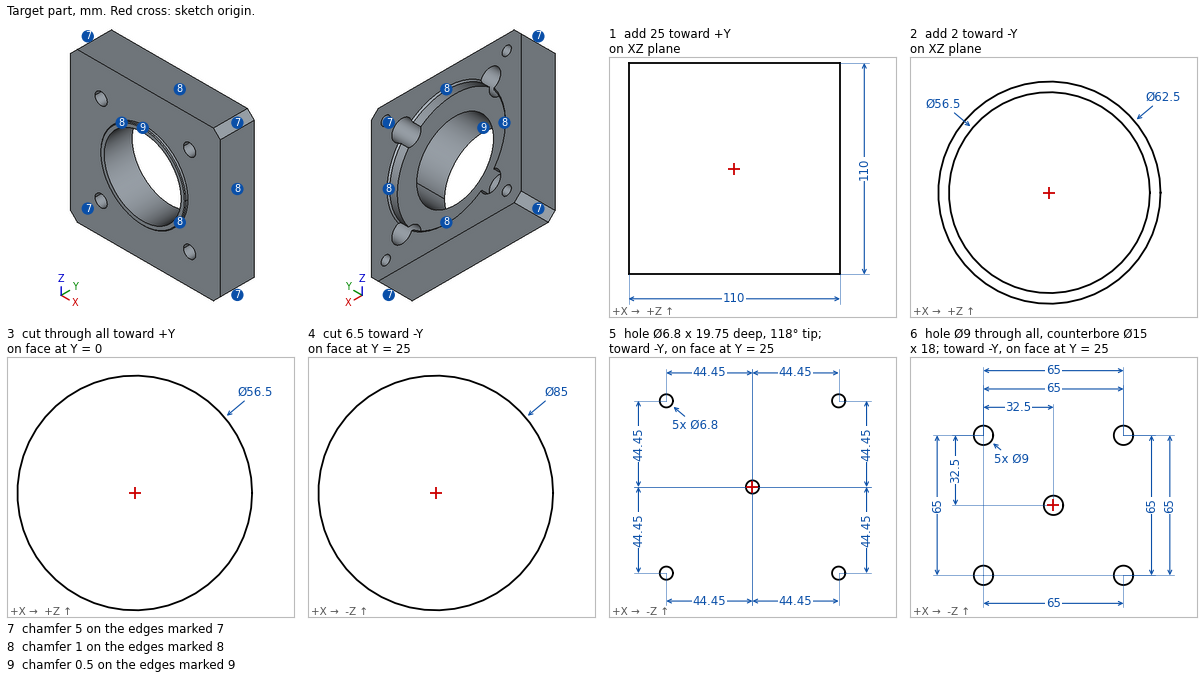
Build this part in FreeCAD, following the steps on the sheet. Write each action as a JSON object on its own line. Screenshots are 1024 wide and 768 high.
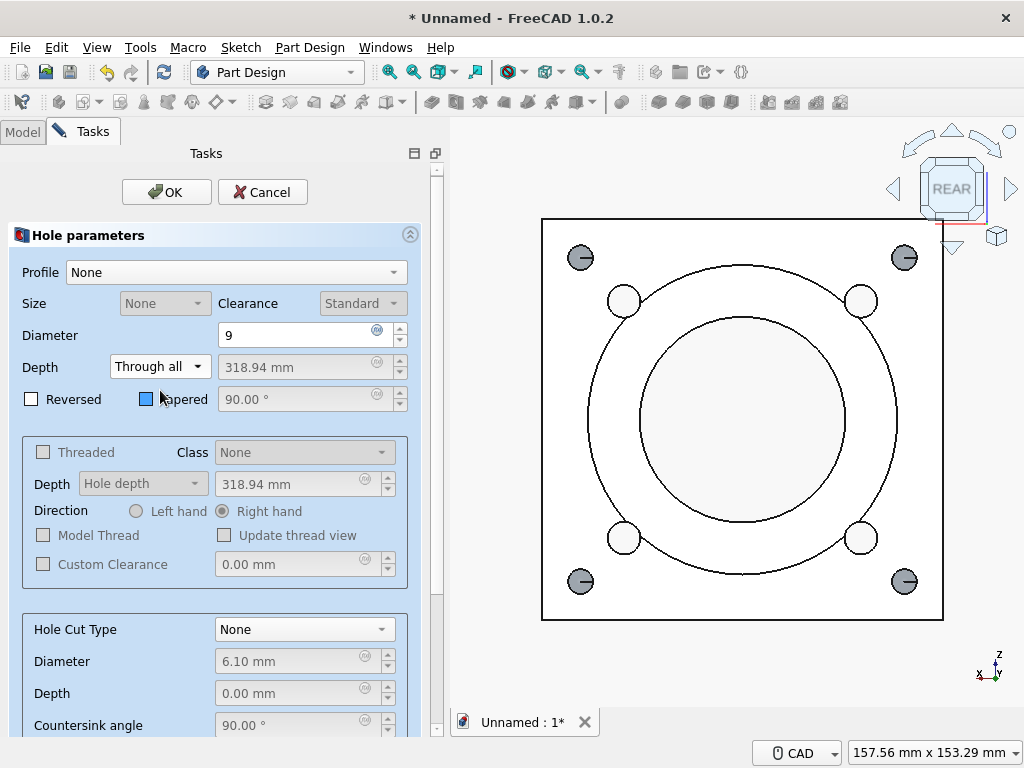
{"action": "left_click", "coordinate": [306, 630]}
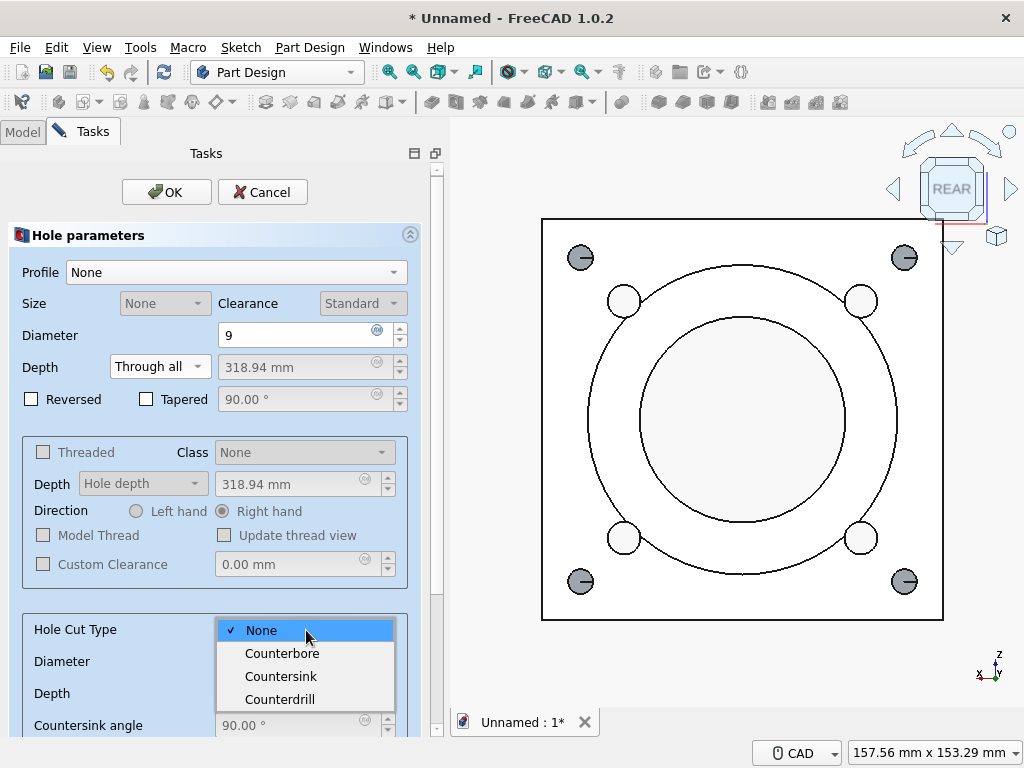
{"action": "left_click", "coordinate": [304, 654]}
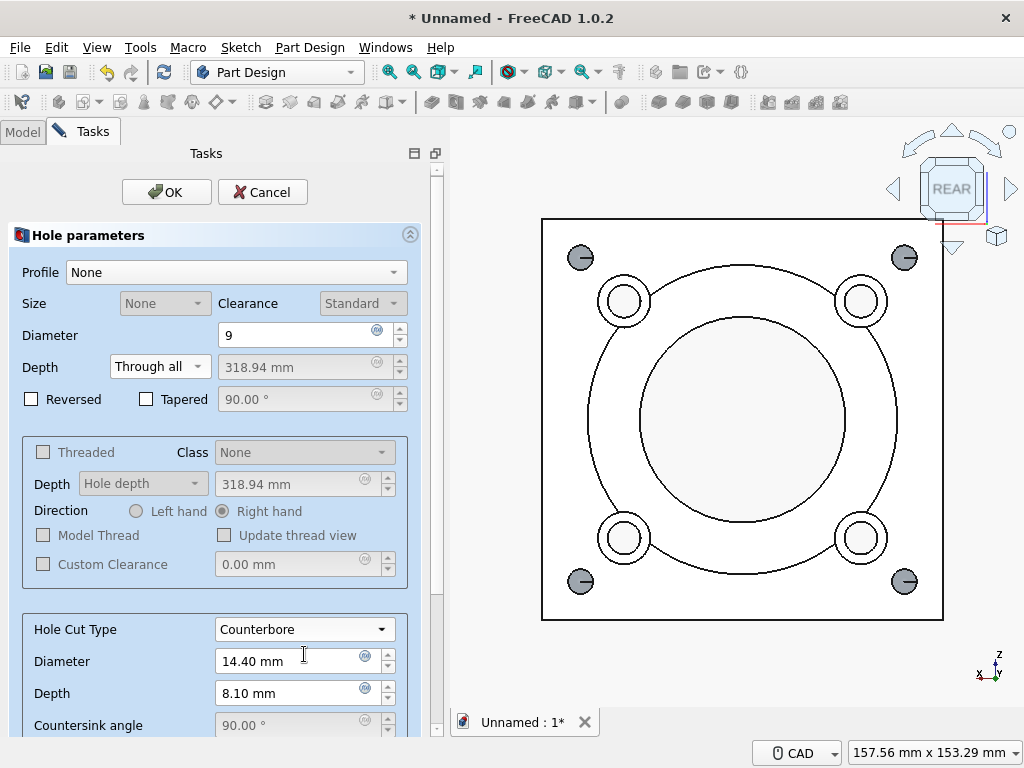
{"action": "triple_click", "coordinate": [298, 661]}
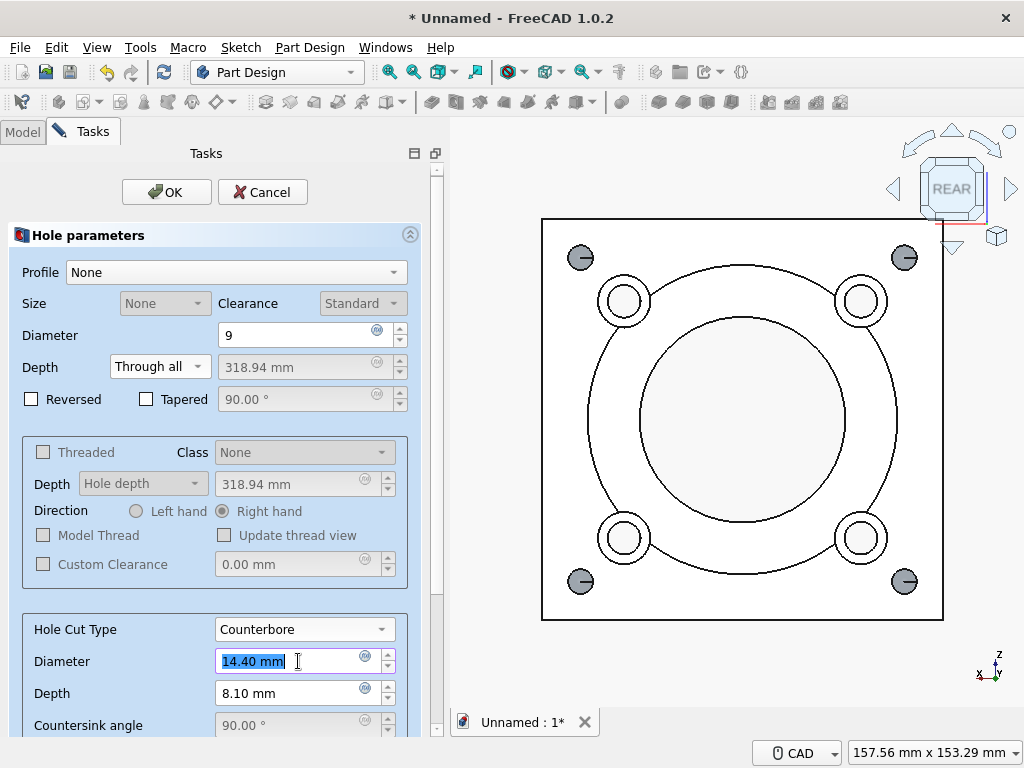
{"action": "type", "text": "15"}
{"action": "key", "text": "Tab"}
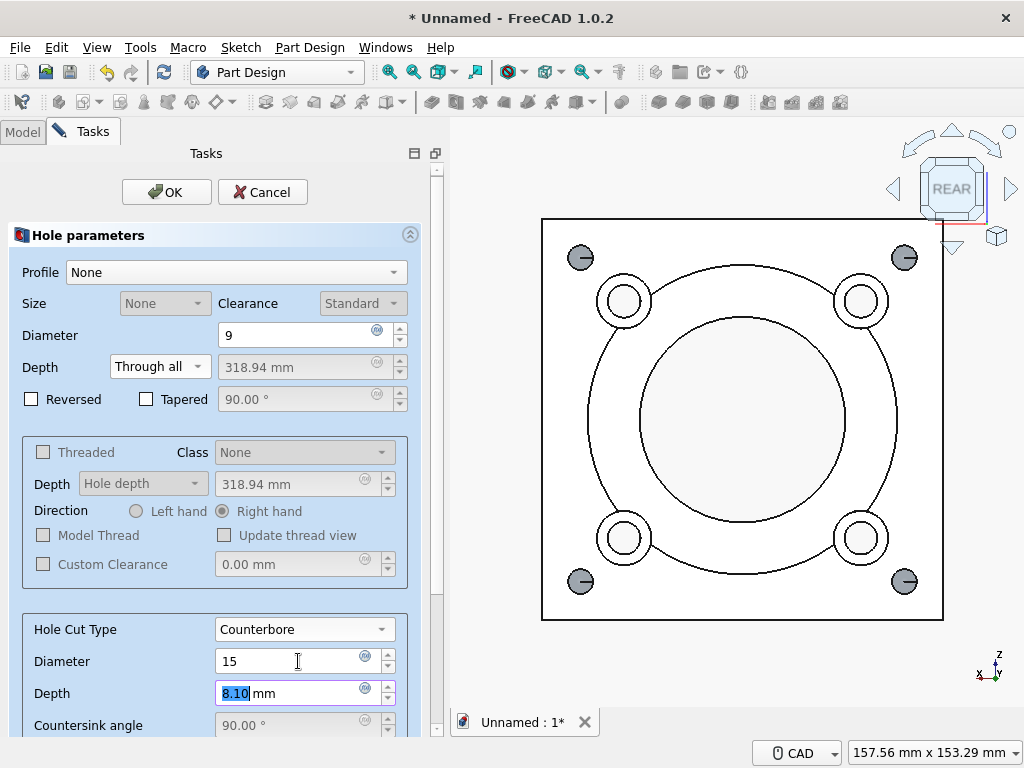
{"action": "type", "text": "18"}
{"action": "key", "text": "Tab"}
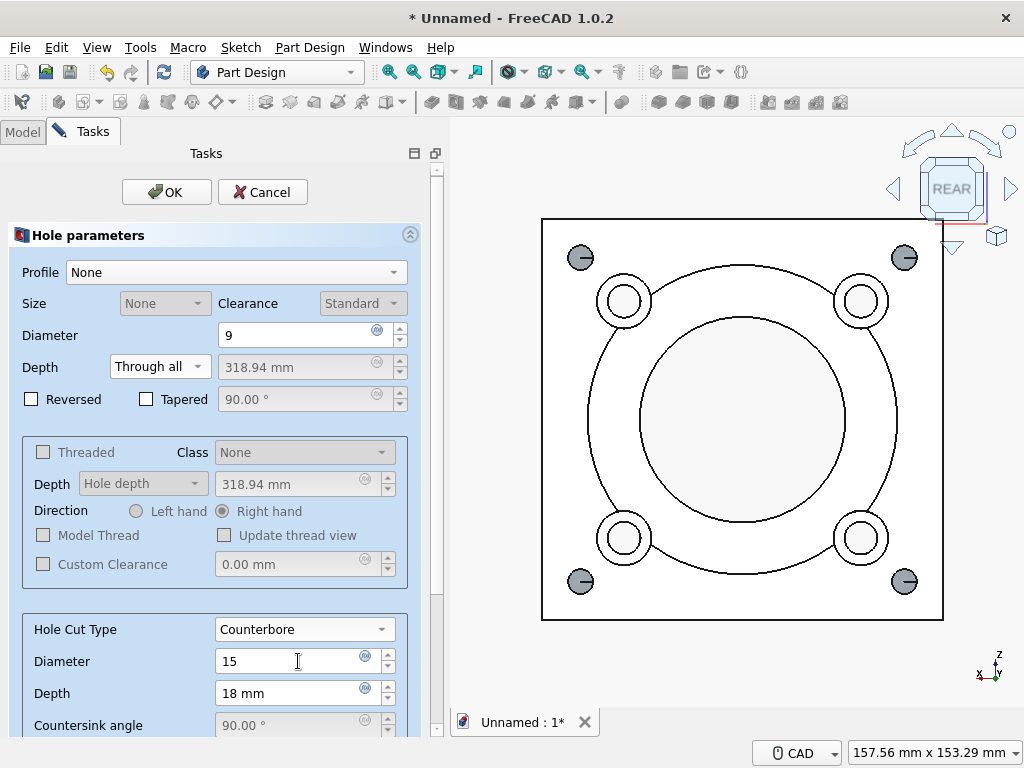
{"action": "left_click", "coordinate": [167, 192]}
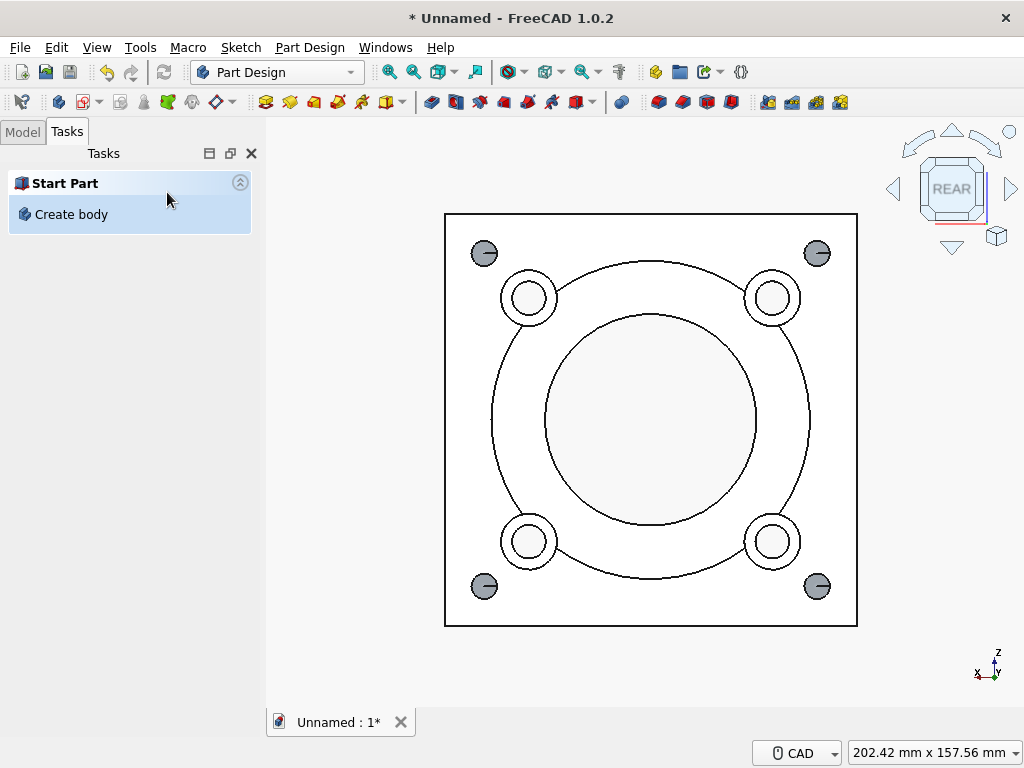
{"action": "key", "text": "0"}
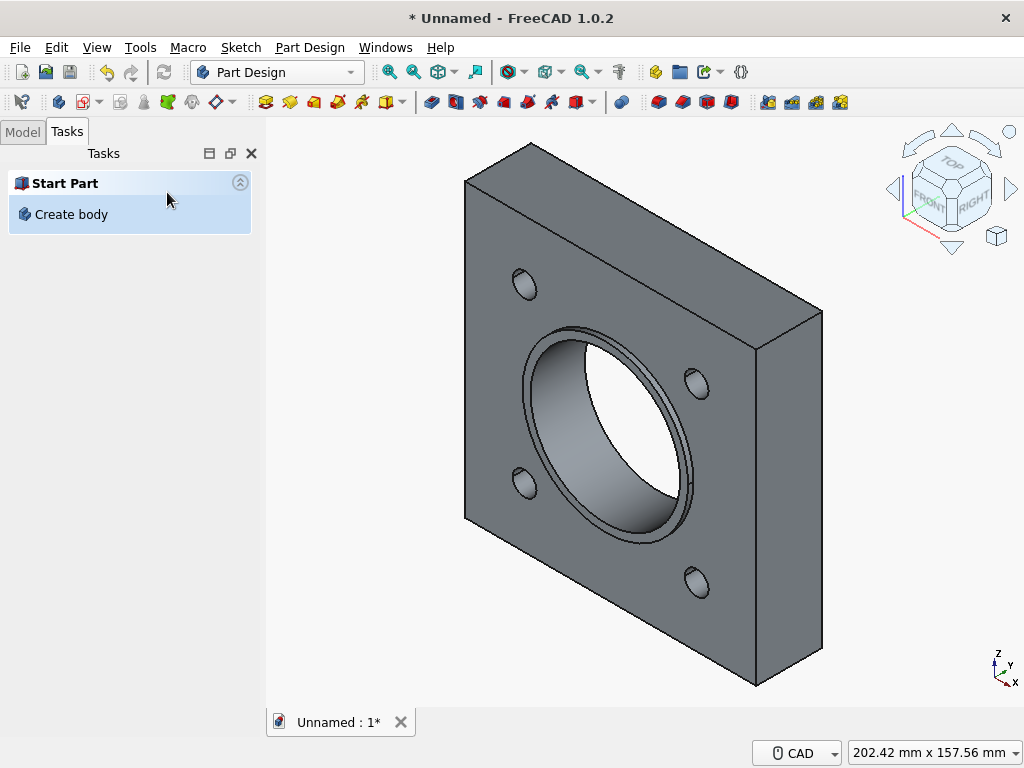
{"action": "left_click", "coordinate": [789, 329]}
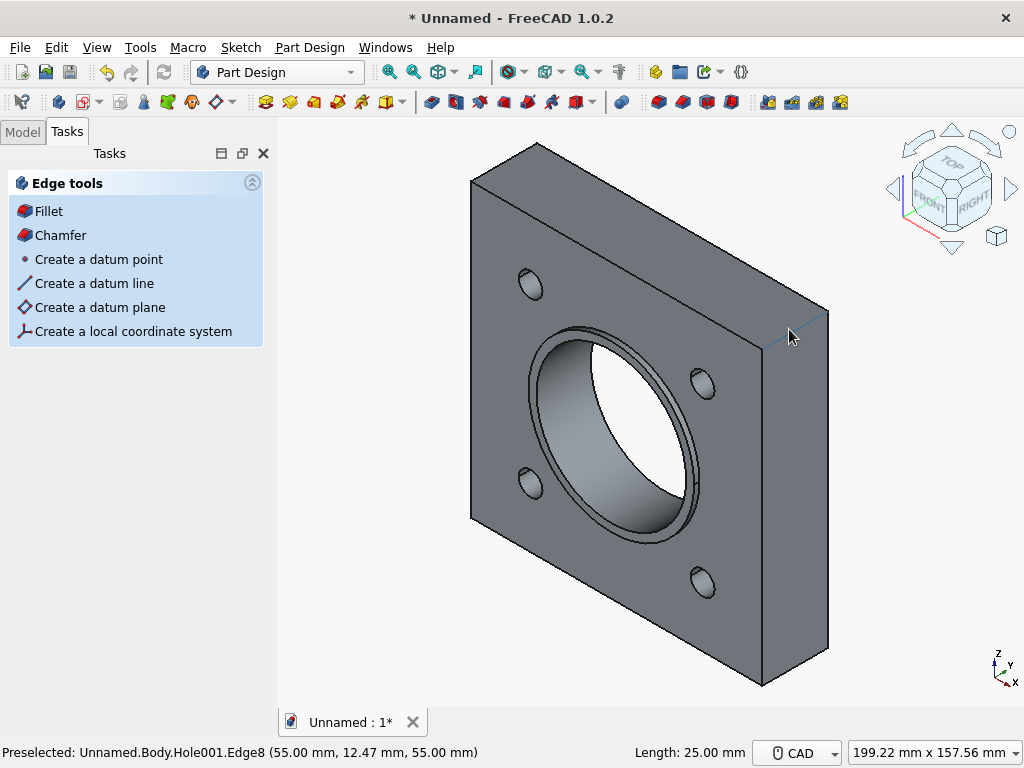
{"action": "key", "text": "2"}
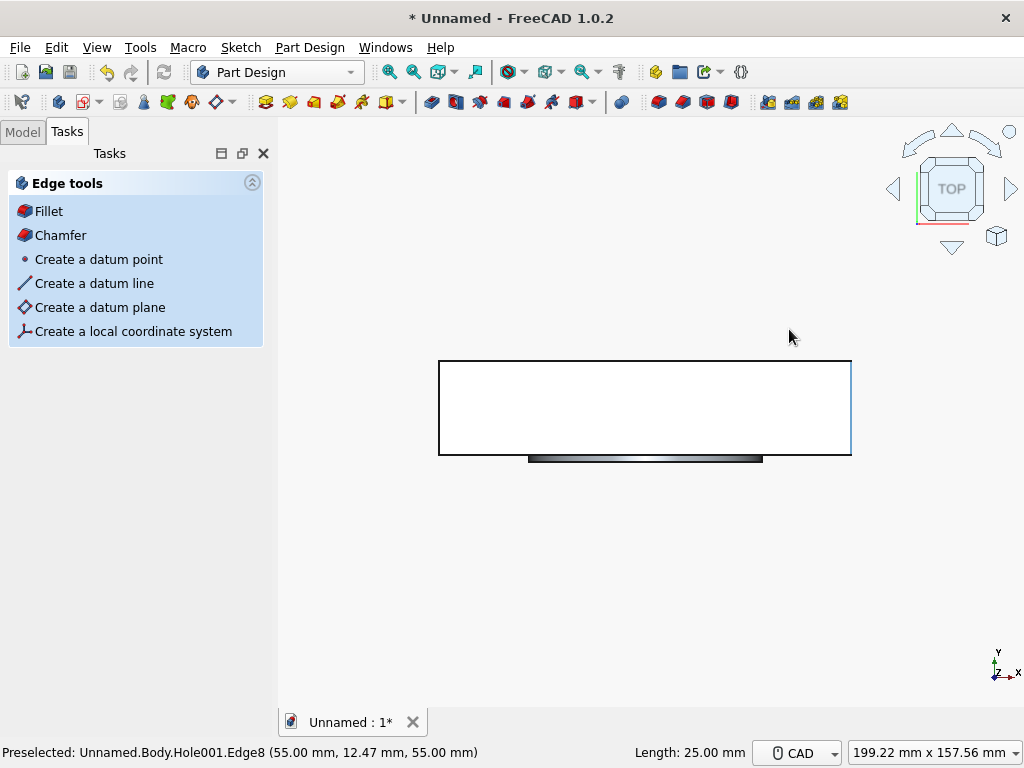
{"action": "left_click", "coordinate": [439, 407], "text": "ctrl"}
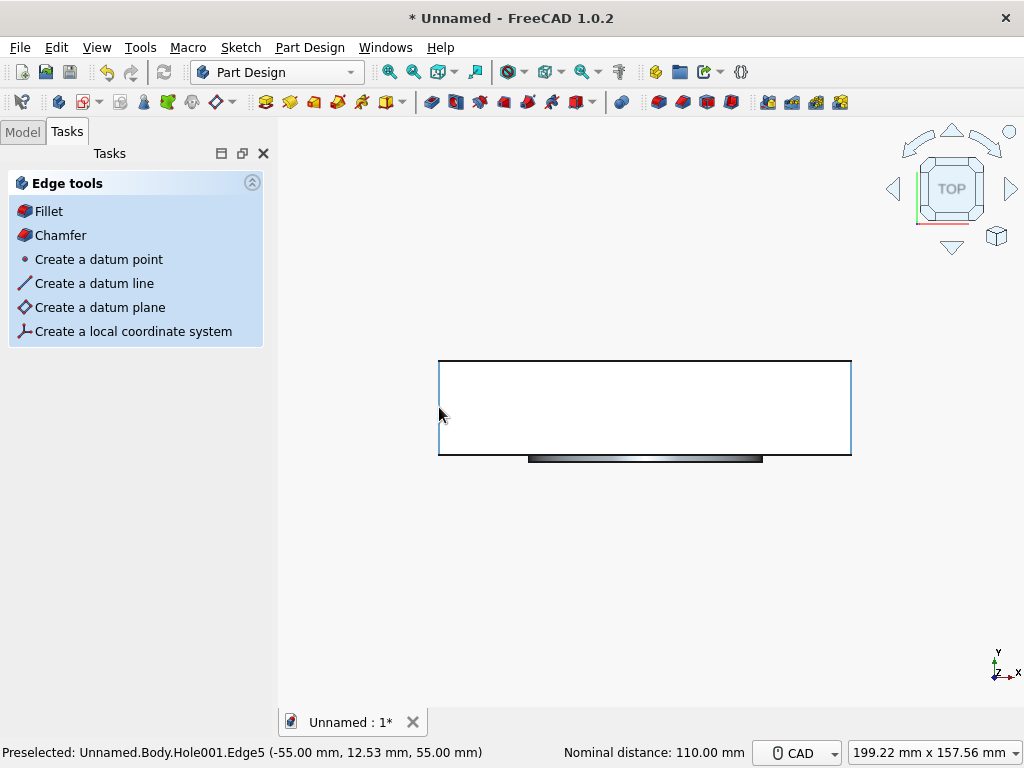
{"action": "key", "text": "1"}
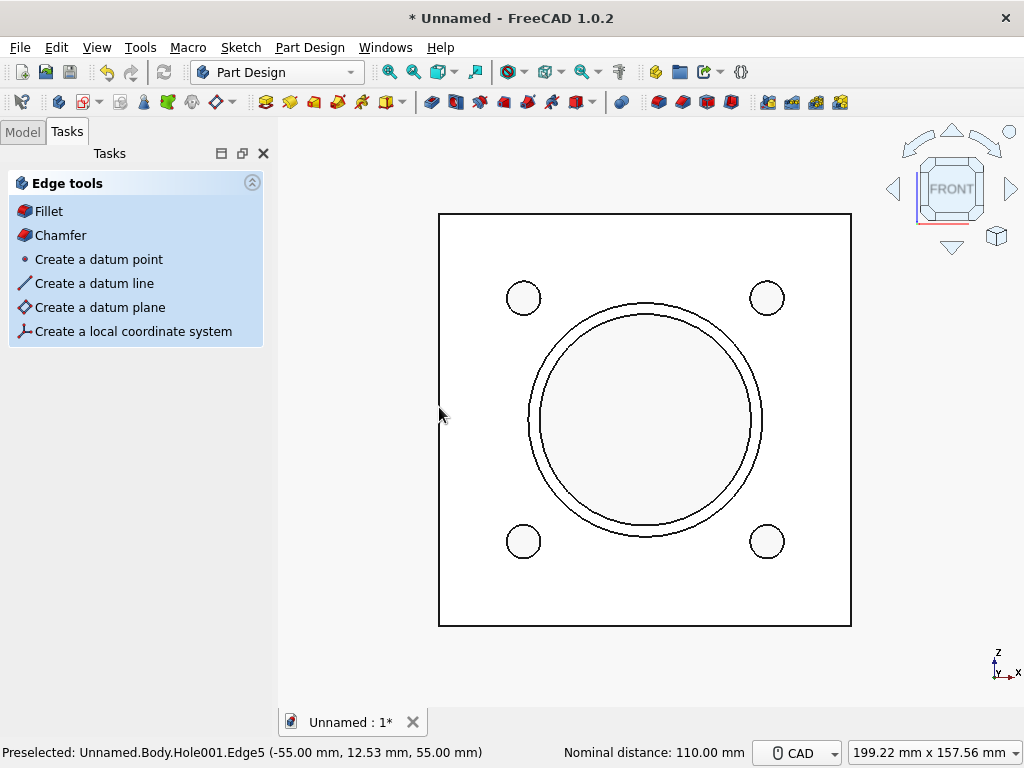
{"action": "key", "text": "3"}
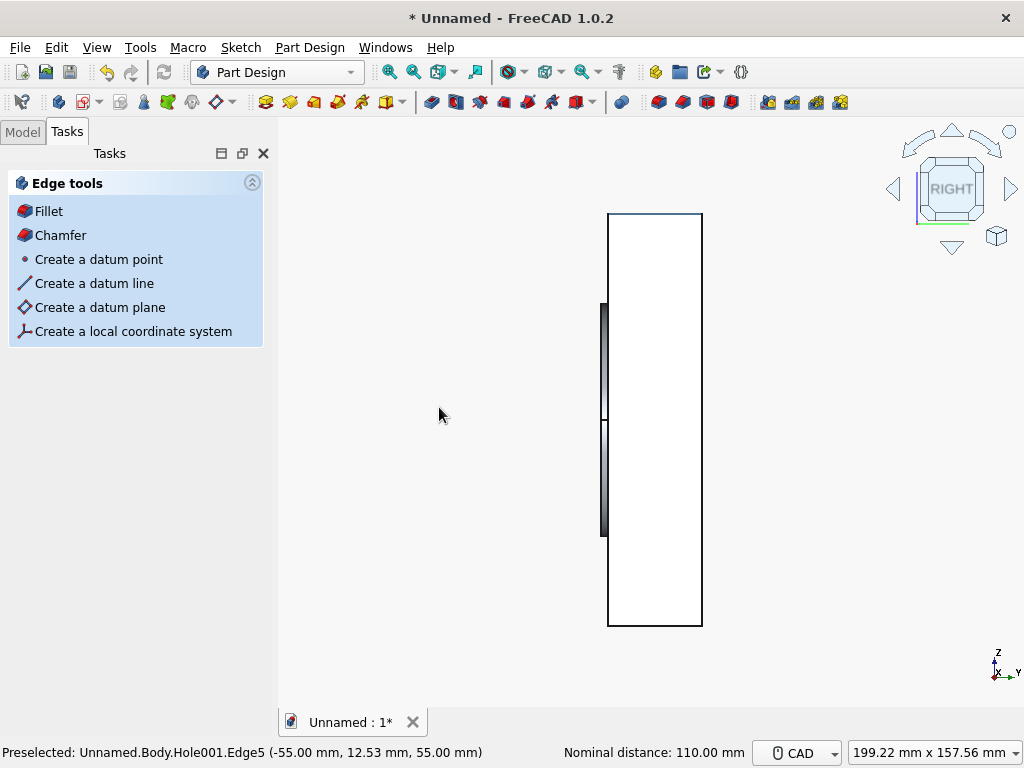
{"action": "left_click", "coordinate": [655, 625], "text": "ctrl"}